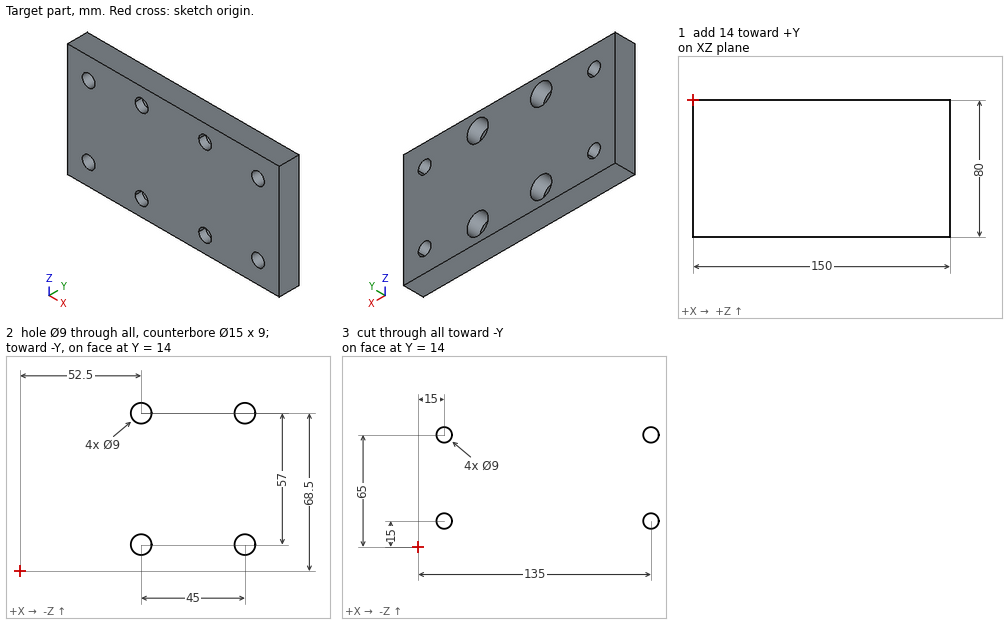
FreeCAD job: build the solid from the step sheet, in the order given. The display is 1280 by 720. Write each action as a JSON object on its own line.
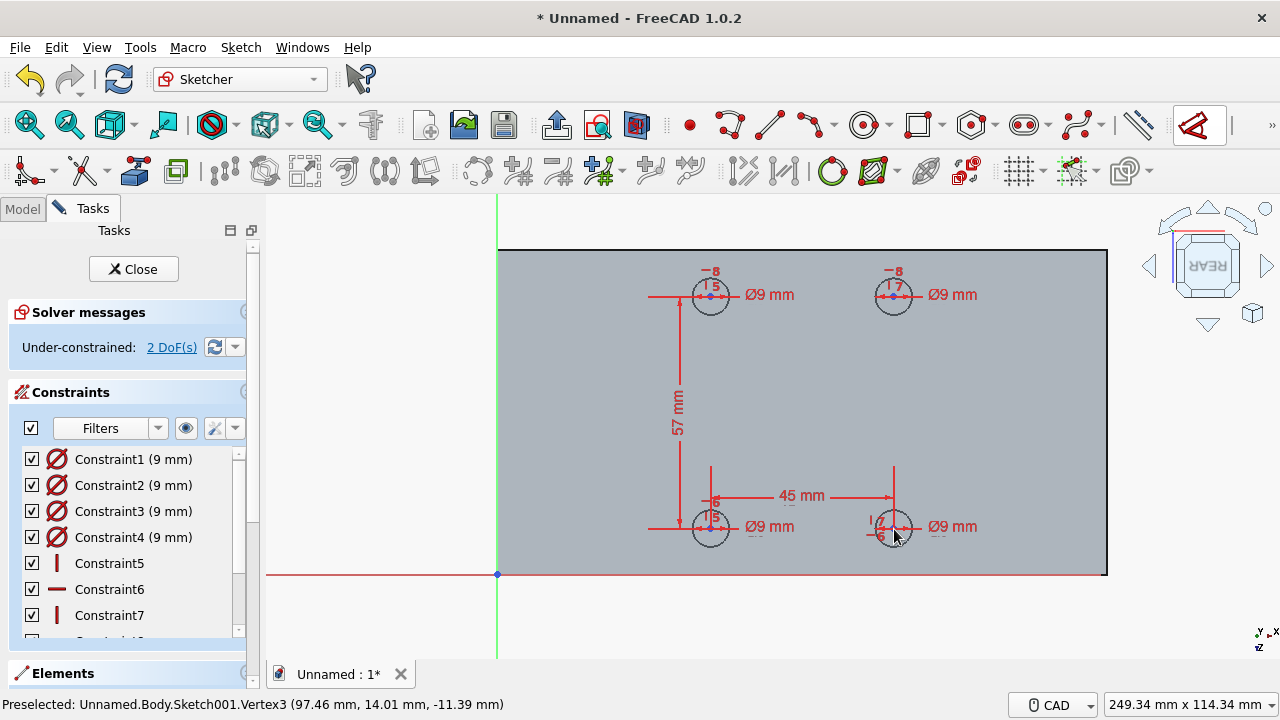
{"action": "left_click", "coordinate": [711, 297]}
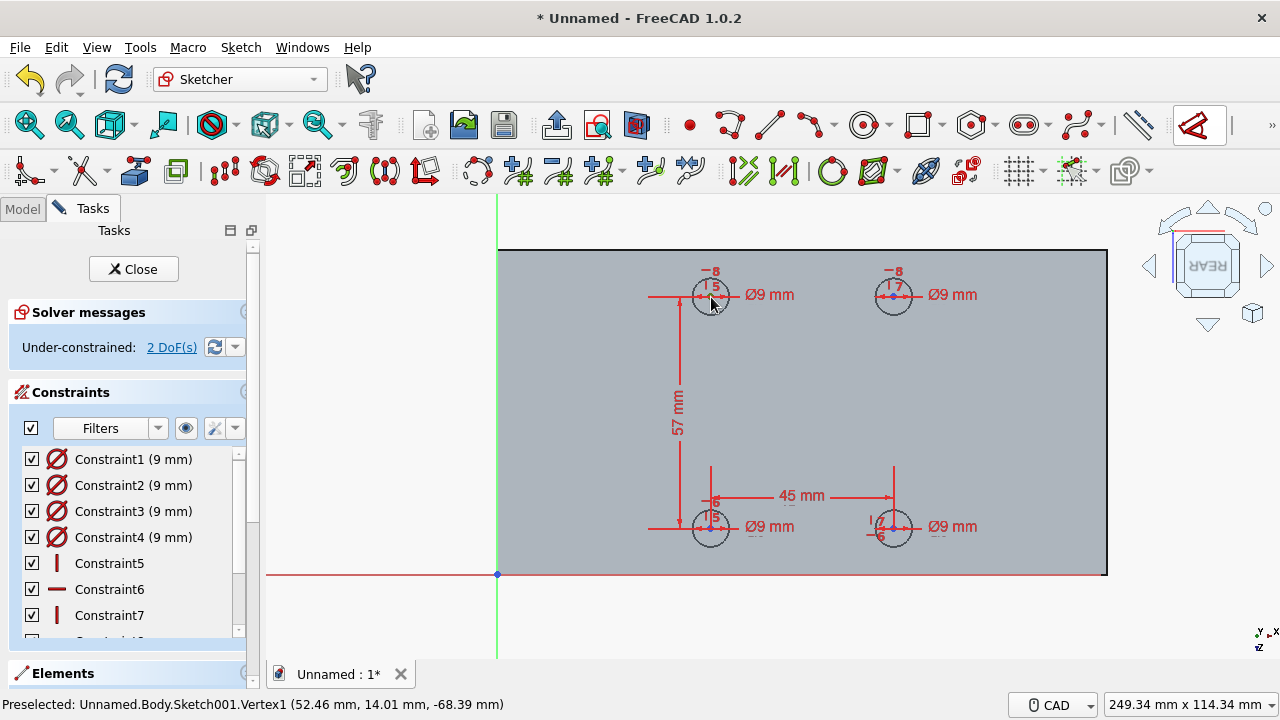
{"action": "key", "text": "l"}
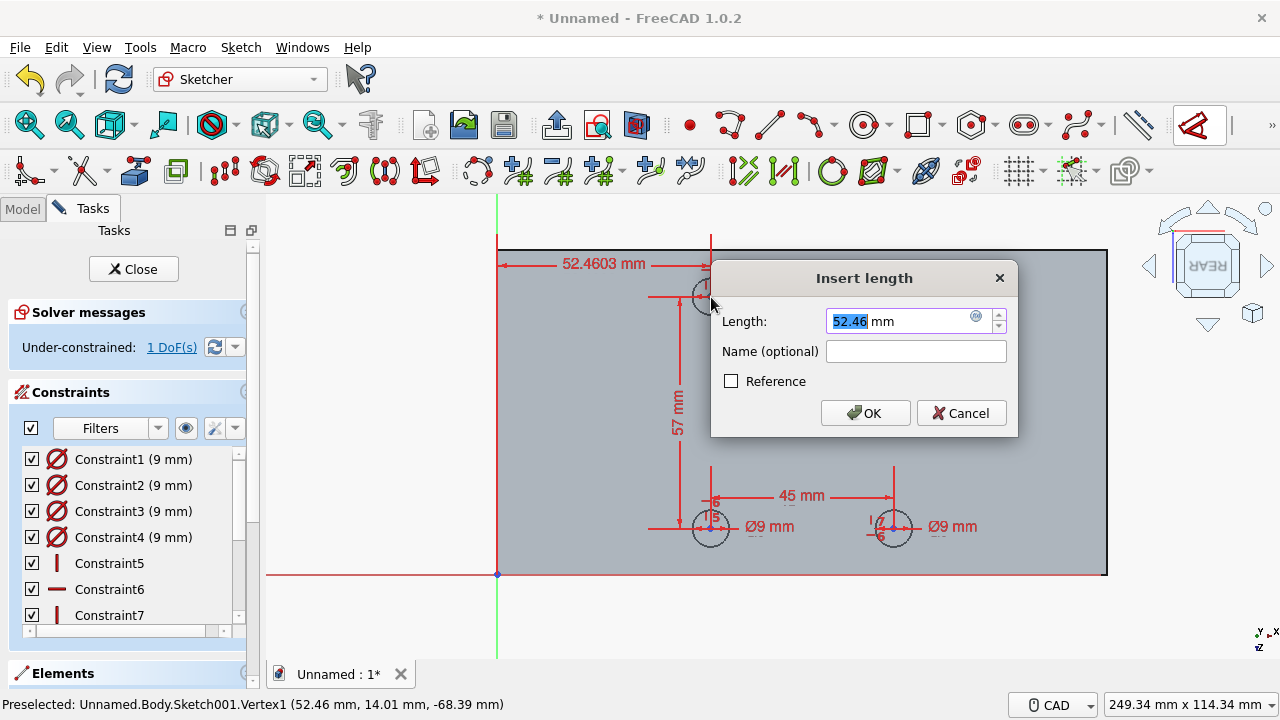
{"action": "type", "text": "52.5"}
{"action": "key", "text": "Return"}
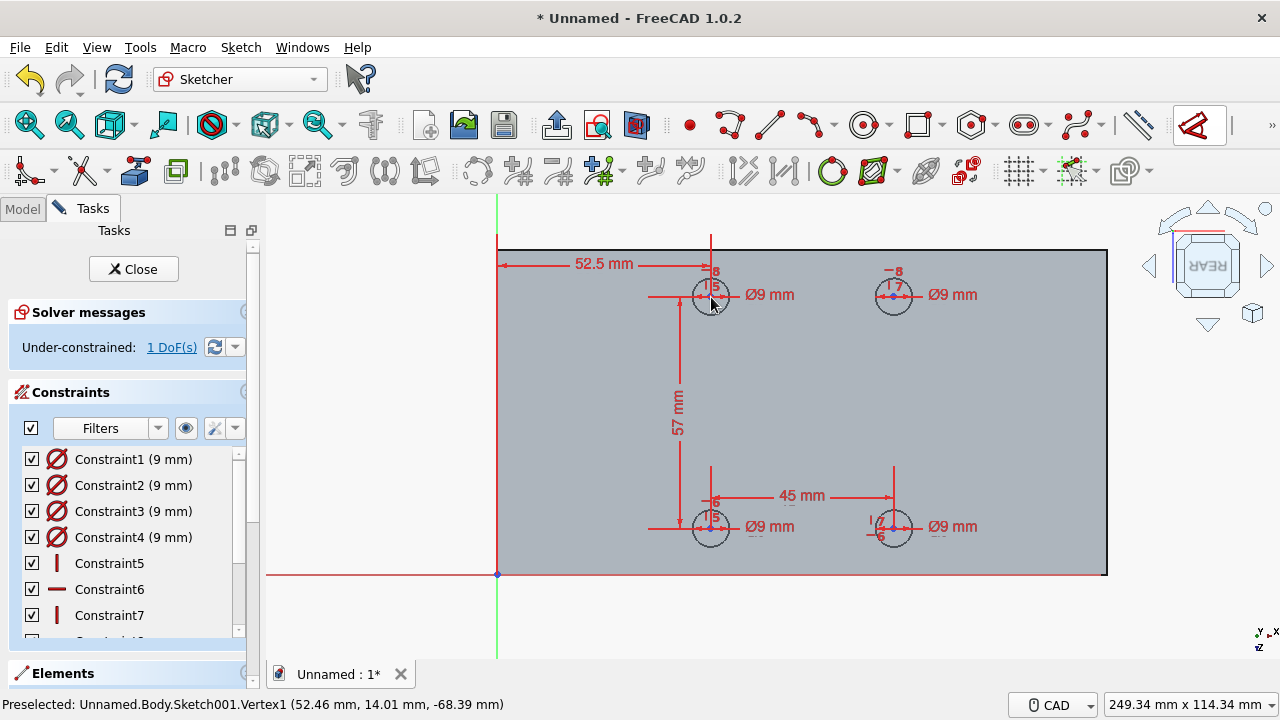
{"action": "left_click", "coordinate": [711, 297]}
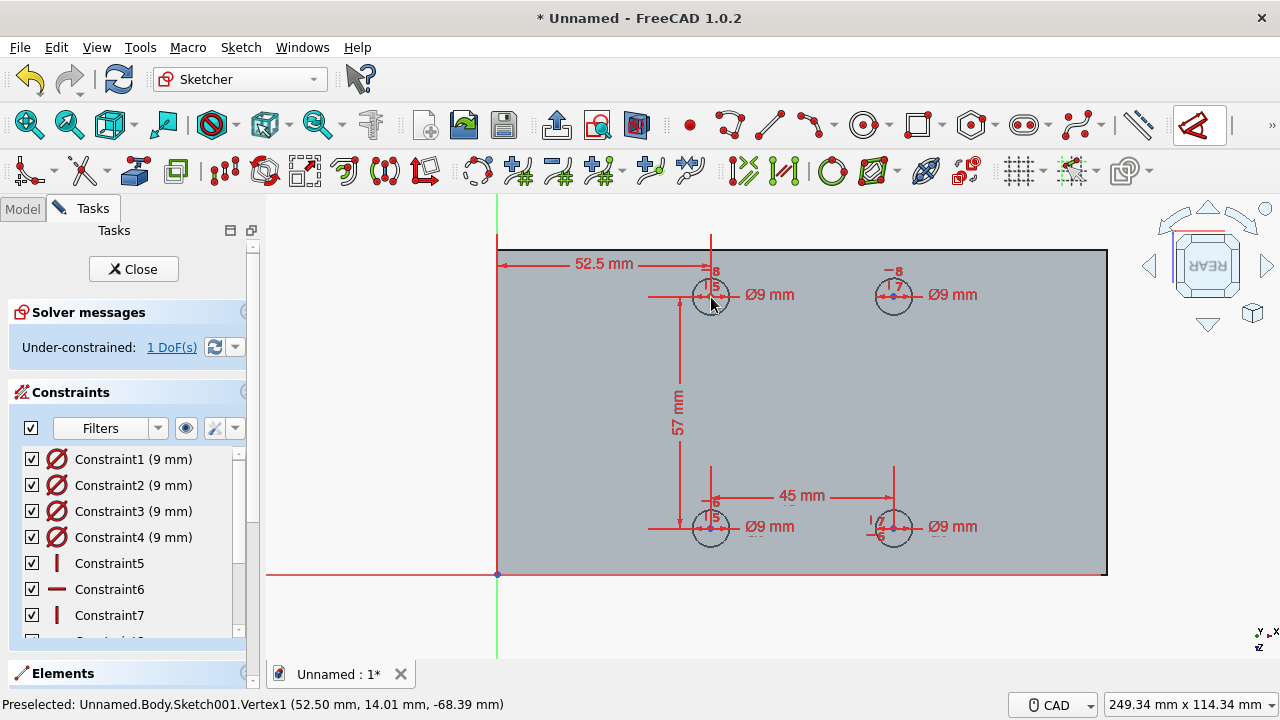
{"action": "left_click", "coordinate": [1220, 126]}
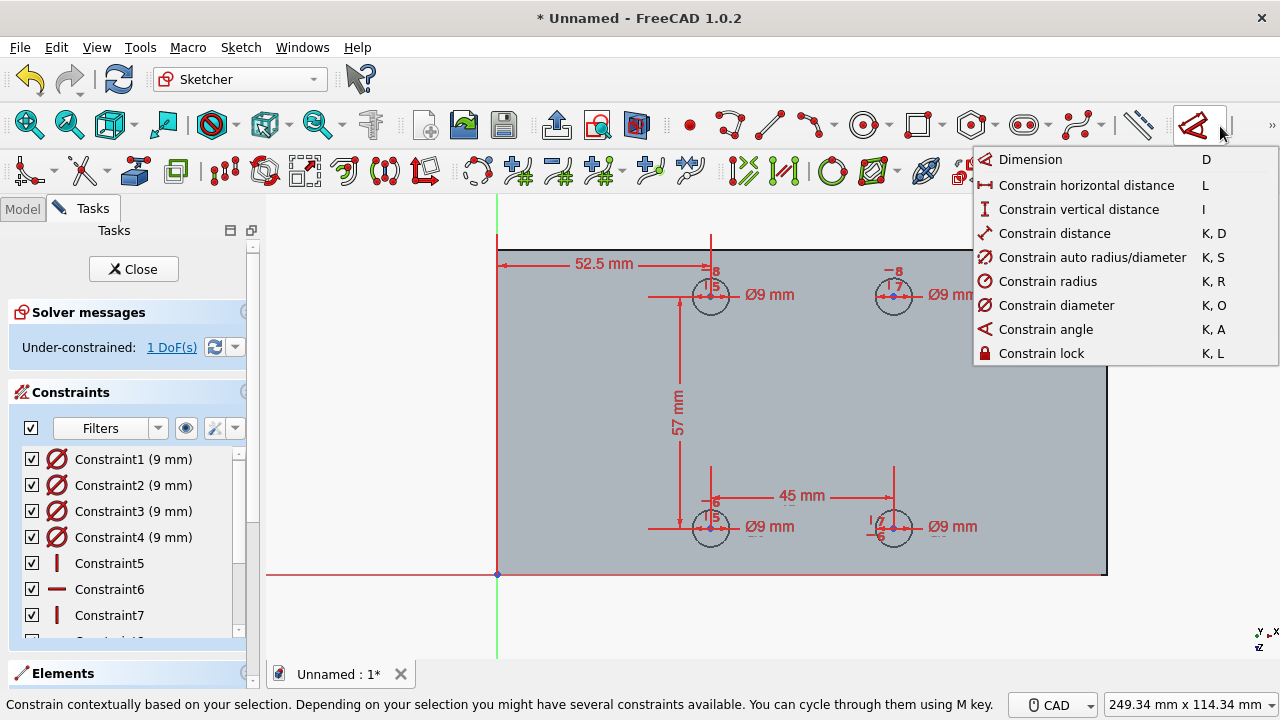
{"action": "left_click", "coordinate": [1126, 209]}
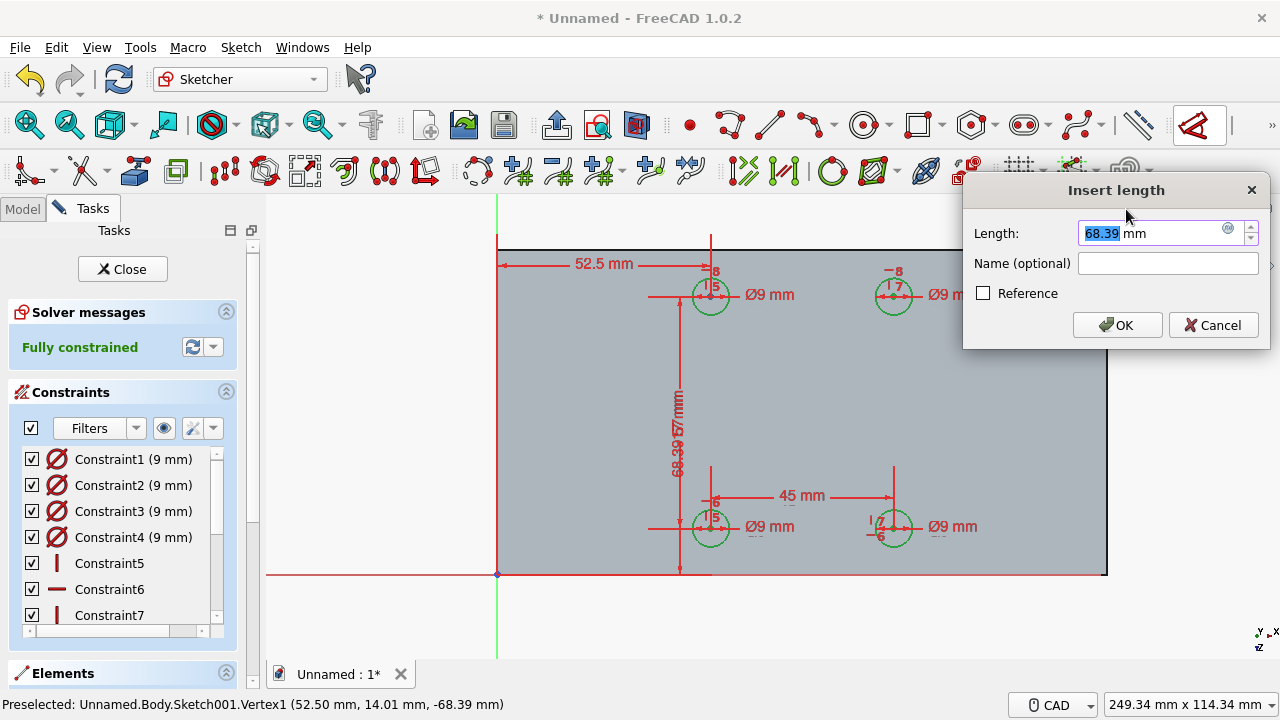
{"action": "type", "text": "68.5"}
{"action": "key", "text": "Return"}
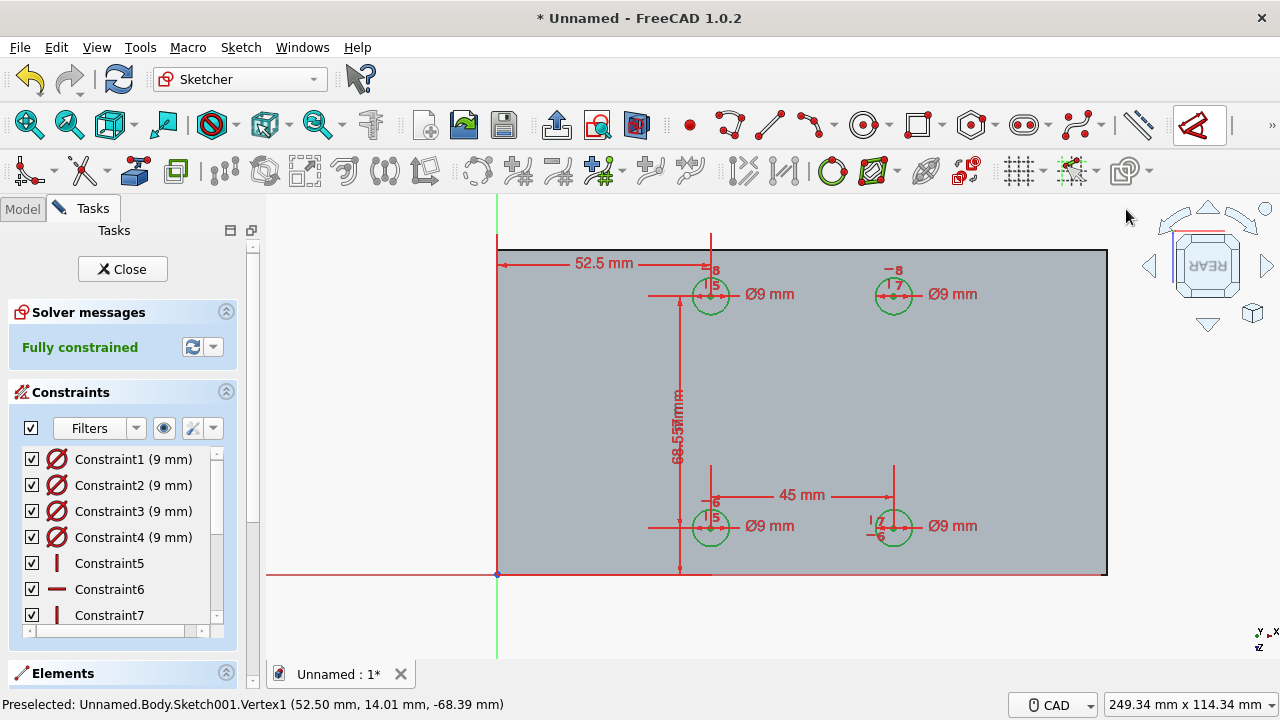
{"action": "left_click", "coordinate": [123, 269]}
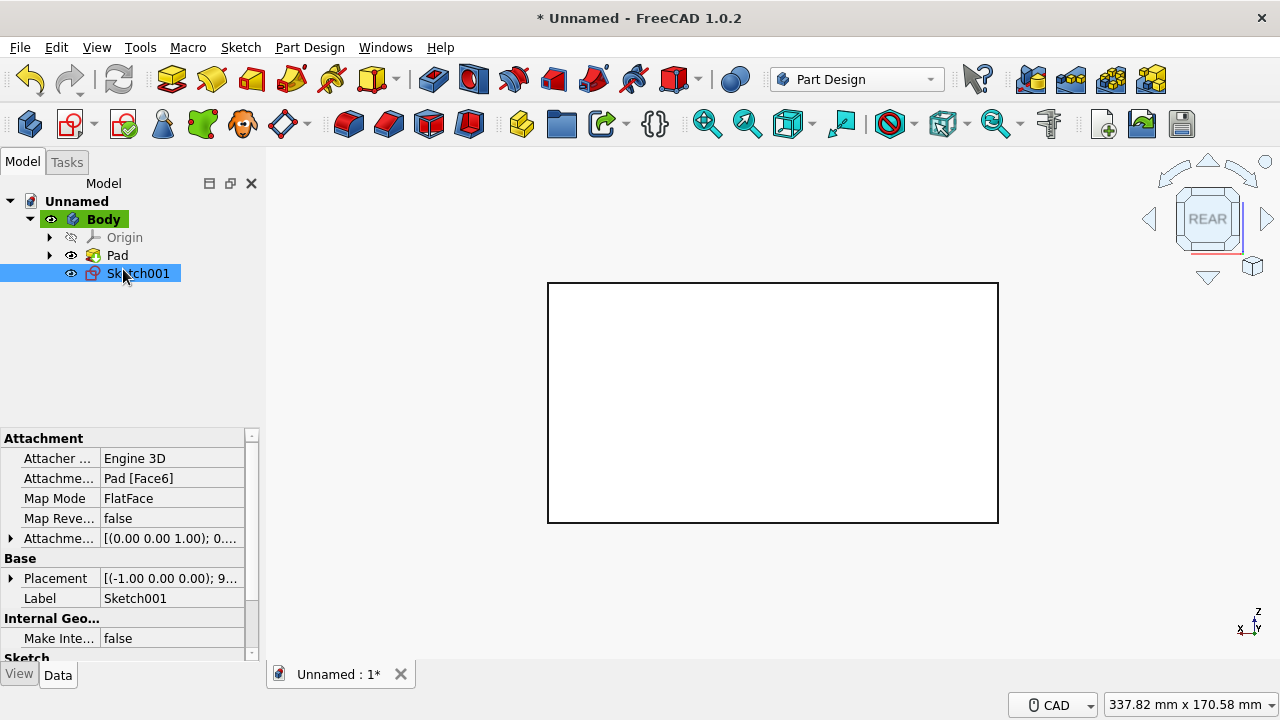
{"action": "left_click", "coordinate": [474, 80]}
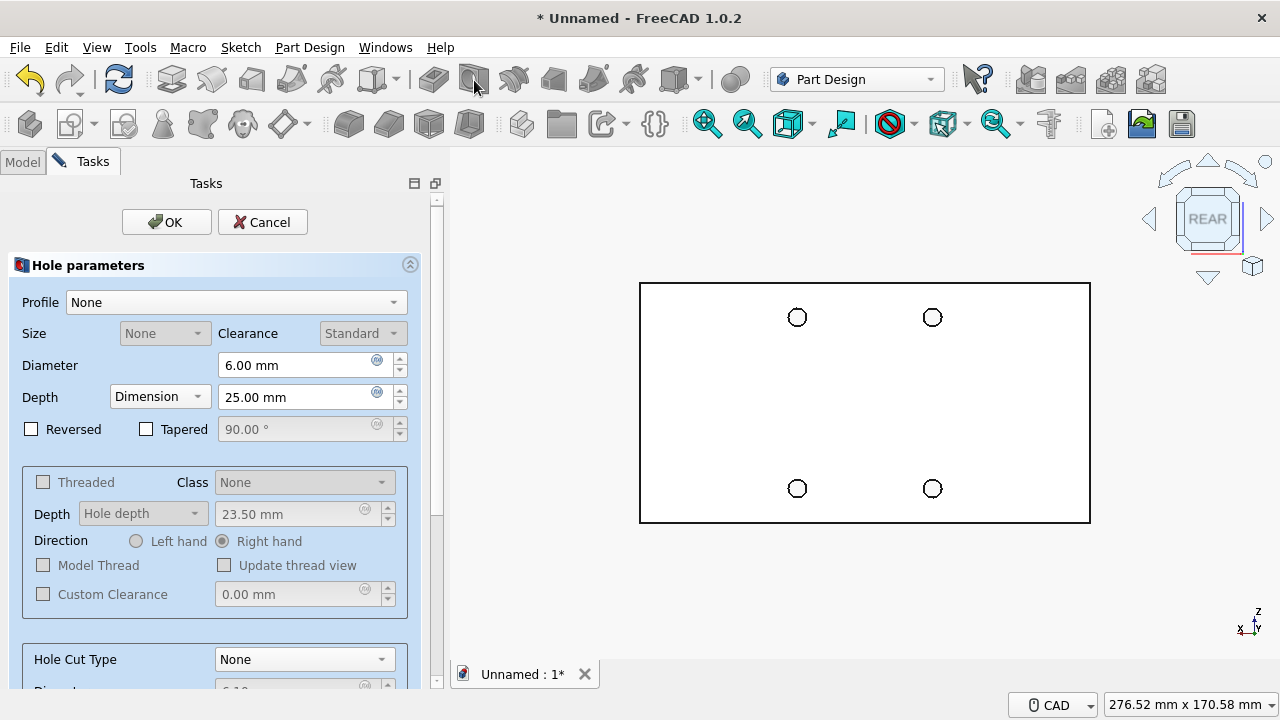
{"action": "triple_click", "coordinate": [305, 365]}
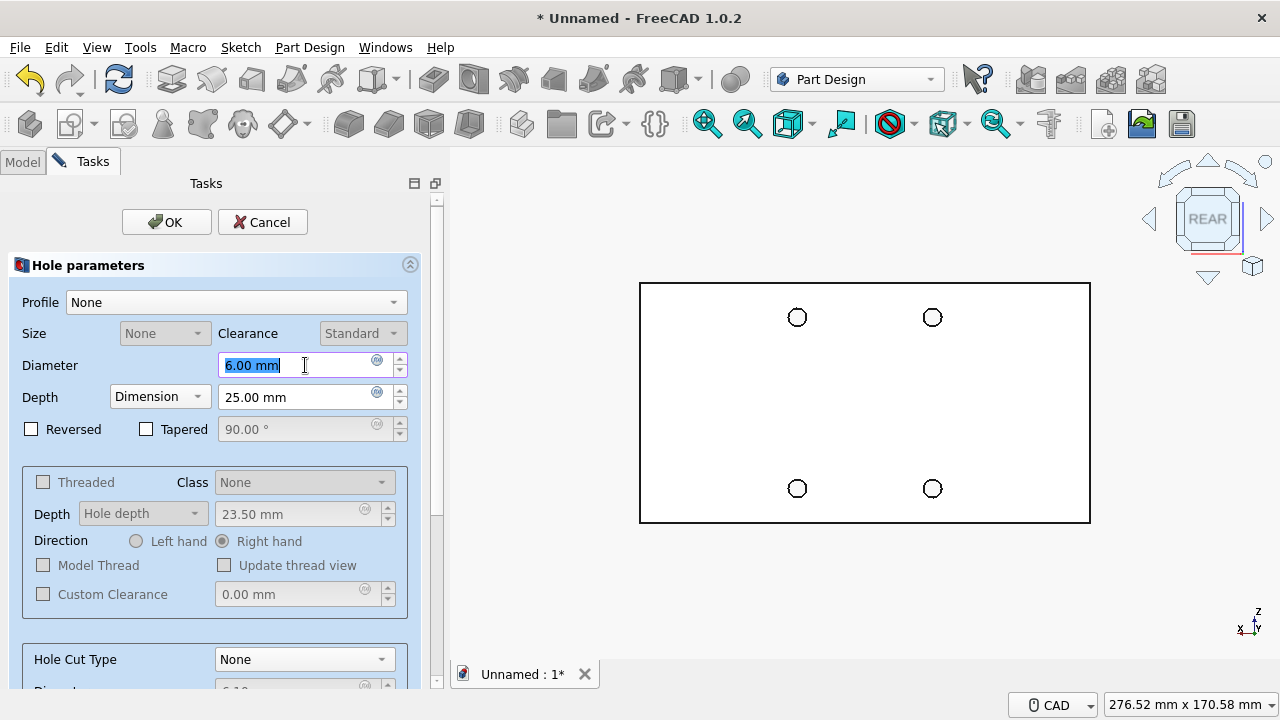
{"action": "type", "text": "9"}
{"action": "key", "text": "Tab"}